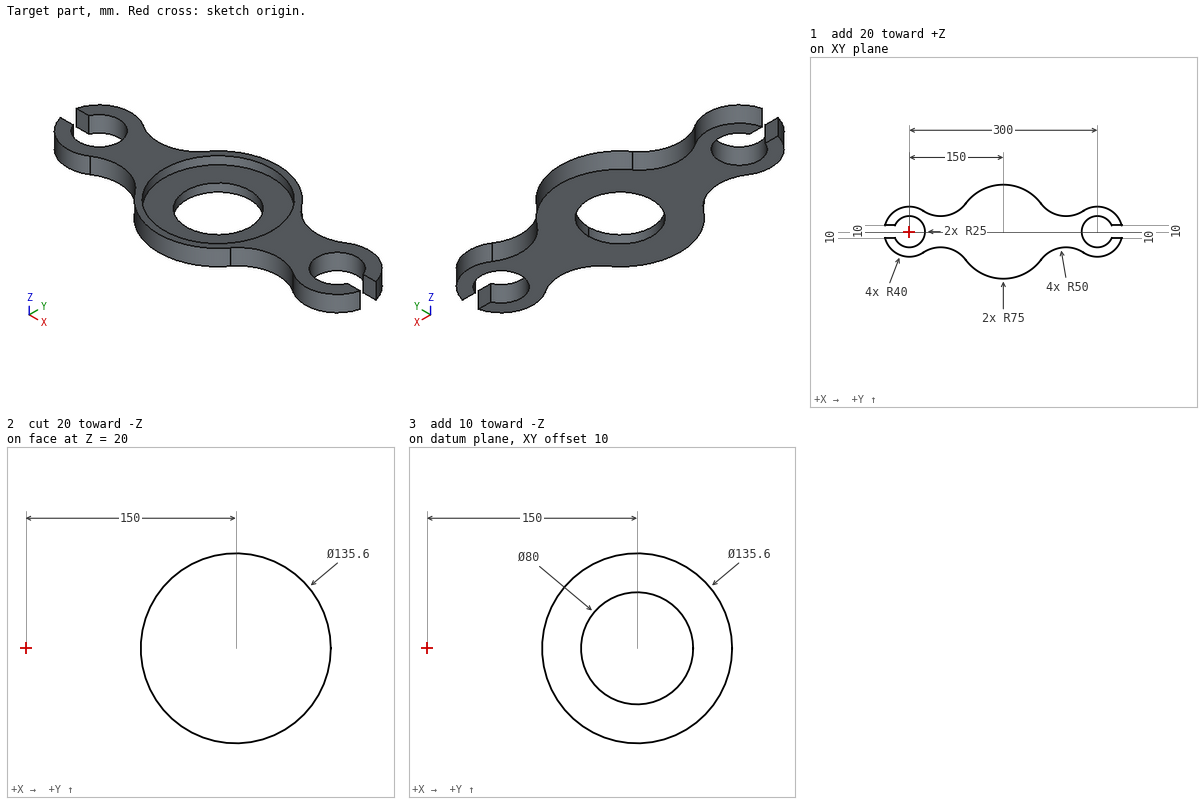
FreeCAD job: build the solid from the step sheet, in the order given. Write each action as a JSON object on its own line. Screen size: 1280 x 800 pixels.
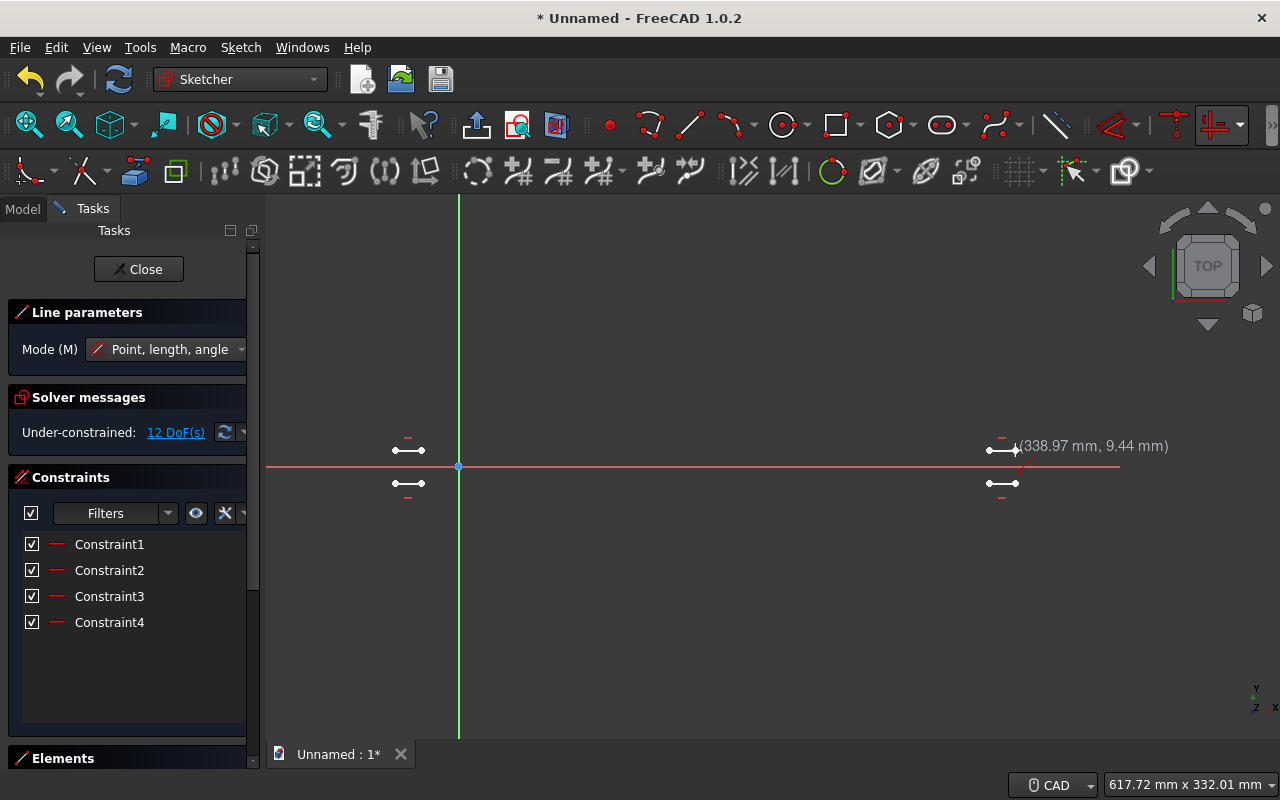
{"action": "left_click", "coordinate": [730, 126]}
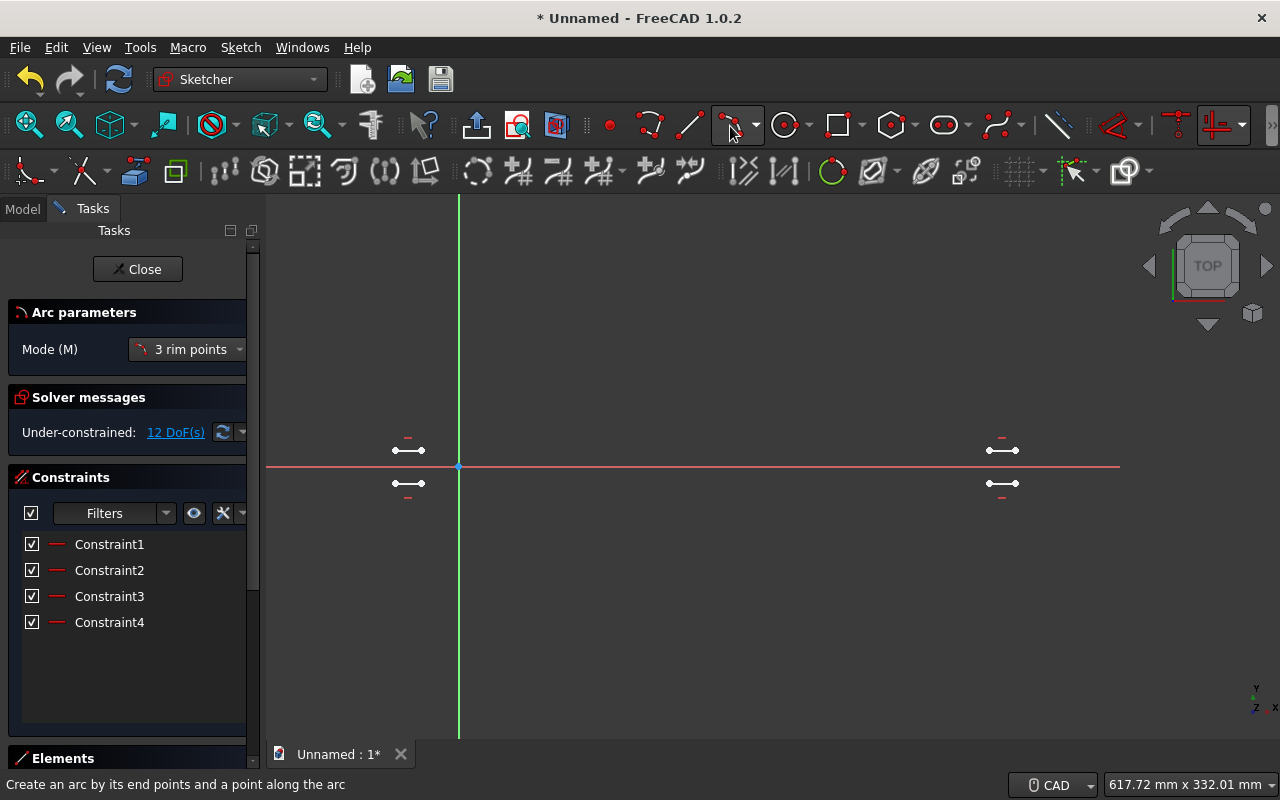
{"action": "scroll", "coordinate": [421, 450], "scroll_direction": "up", "scroll_amount": 2}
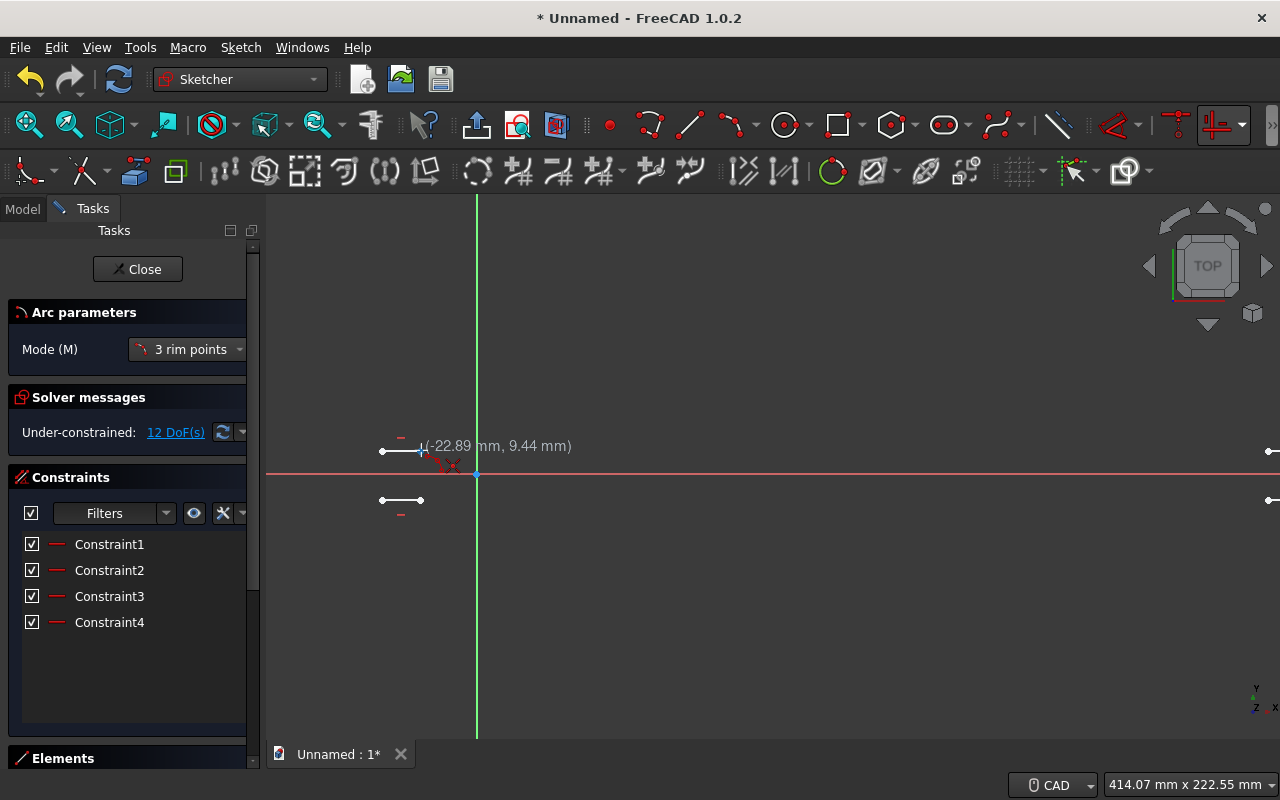
{"action": "left_click", "coordinate": [421, 451]}
{"action": "left_click", "coordinate": [421, 500]}
{"action": "left_click", "coordinate": [529, 506]}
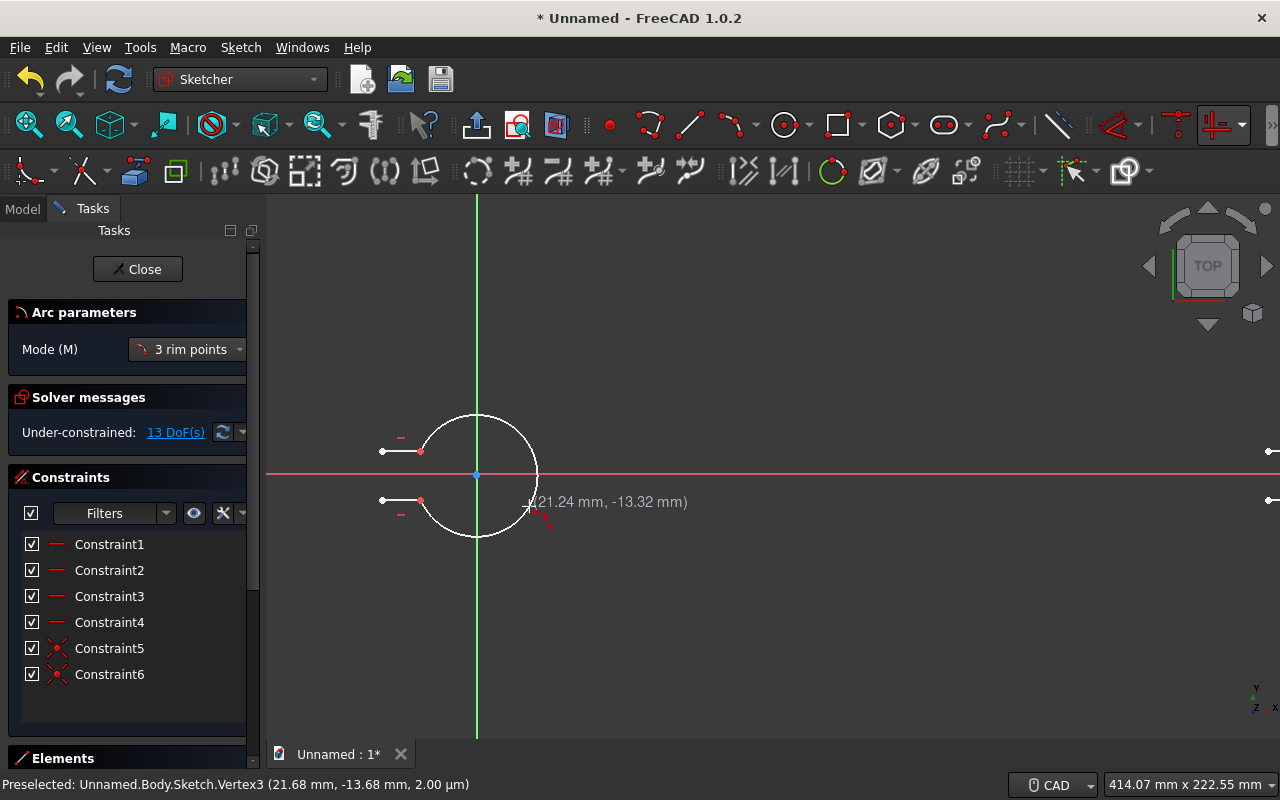
{"action": "left_click", "coordinate": [382, 500]}
{"action": "left_click", "coordinate": [531, 556]}
{"action": "left_click", "coordinate": [442, 566]}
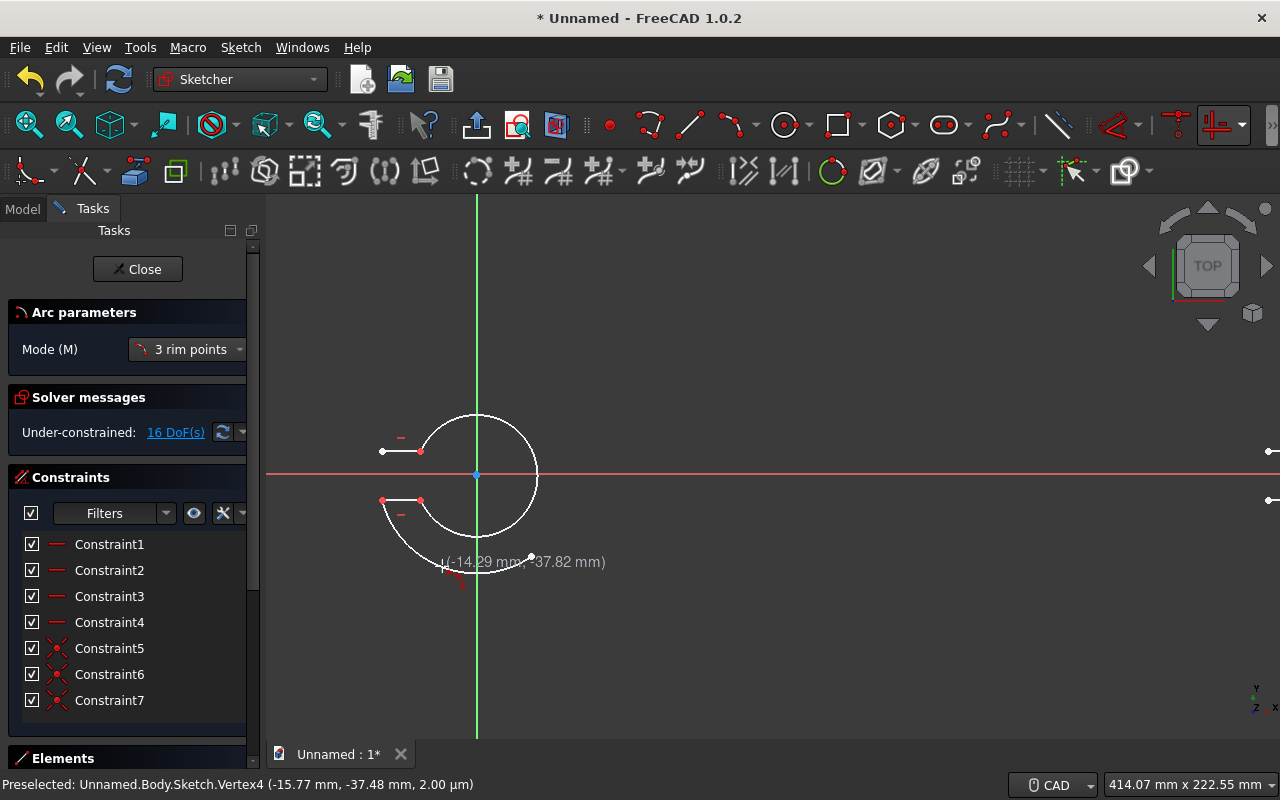
{"action": "left_click", "coordinate": [531, 557]}
{"action": "left_click", "coordinate": [697, 584]}
{"action": "left_click", "coordinate": [620, 537]}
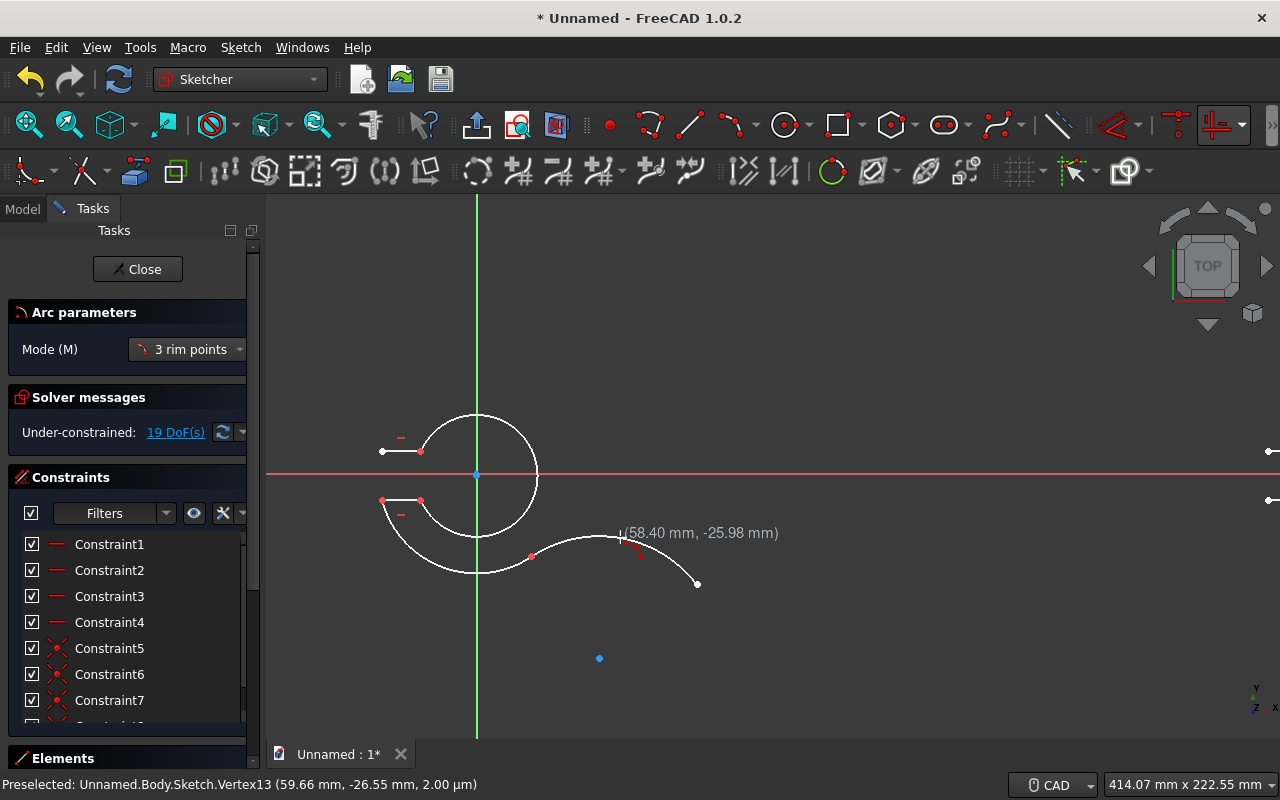
{"action": "left_click", "coordinate": [697, 585]}
{"action": "left_click", "coordinate": [991, 584]}
{"action": "left_click", "coordinate": [844, 658]}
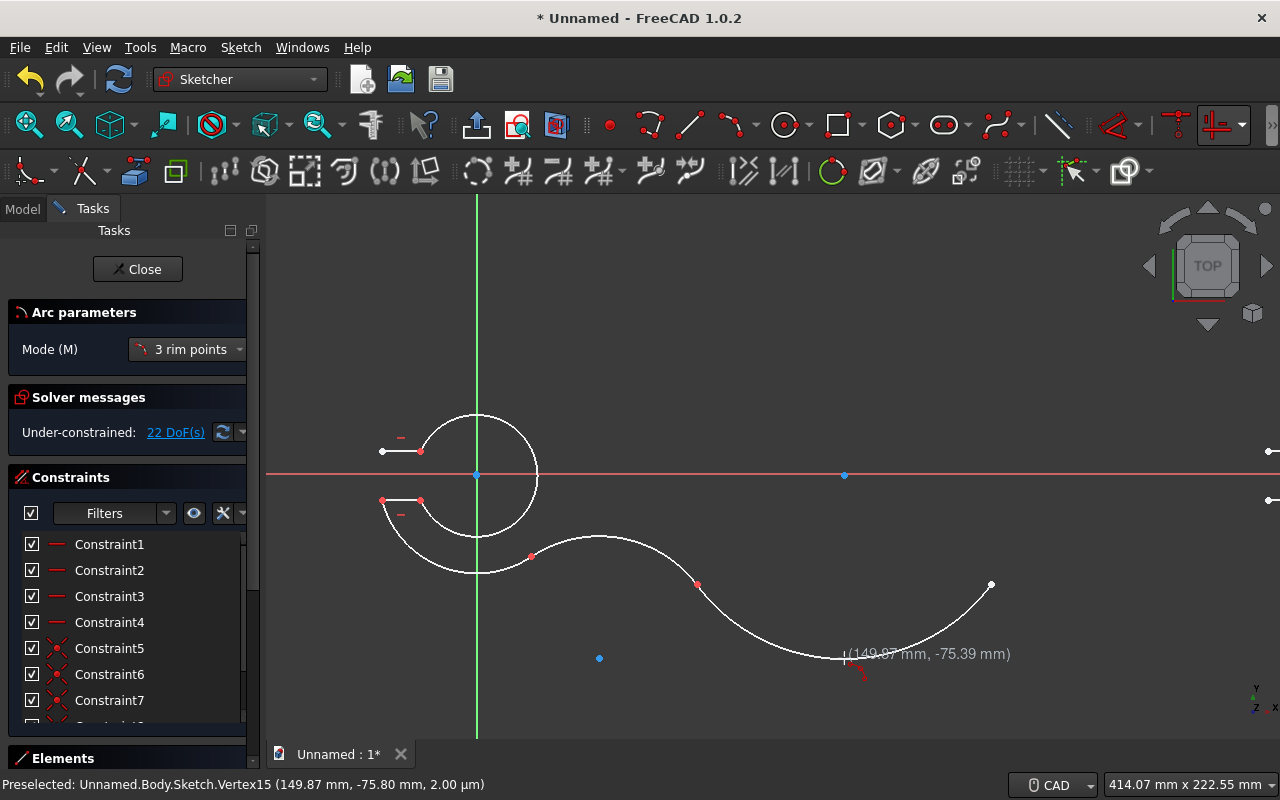
{"action": "left_click", "coordinate": [991, 585]}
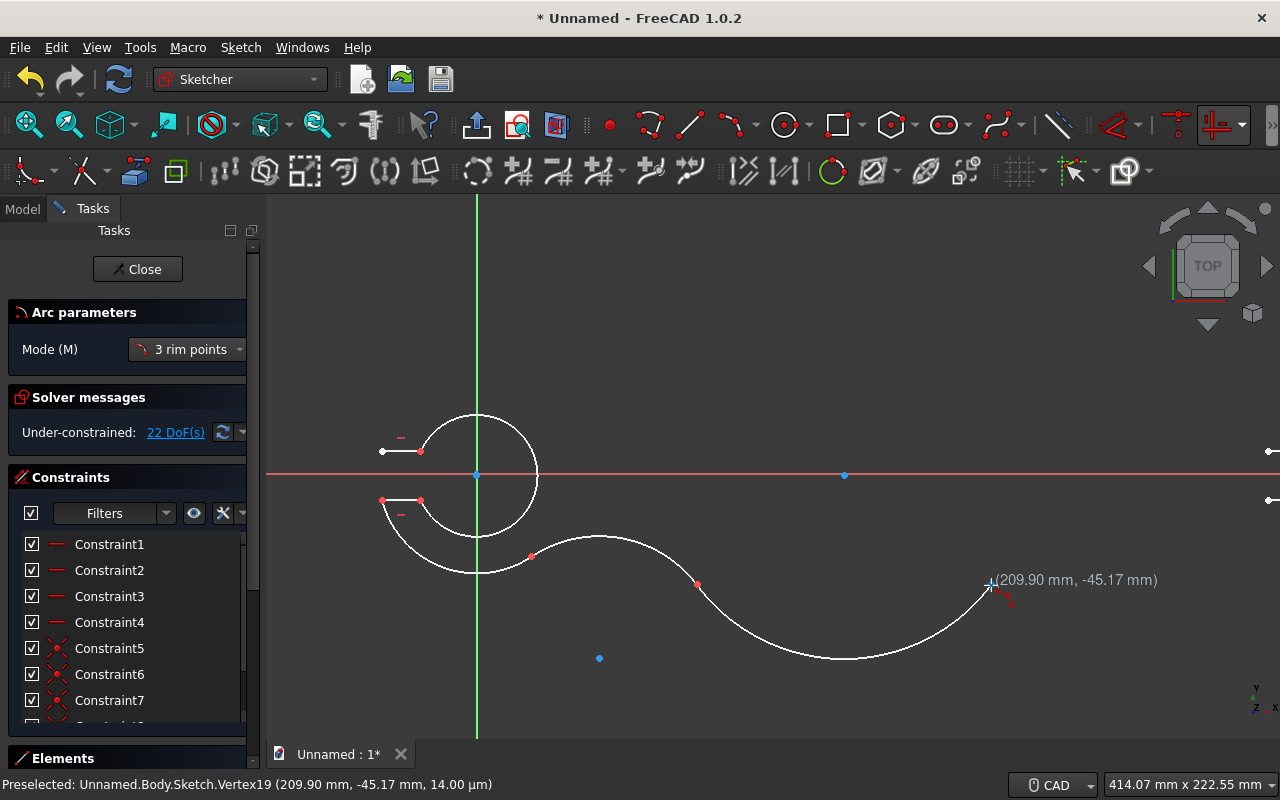
{"action": "scroll", "coordinate": [420, 450], "scroll_direction": "down", "scroll_amount": 2}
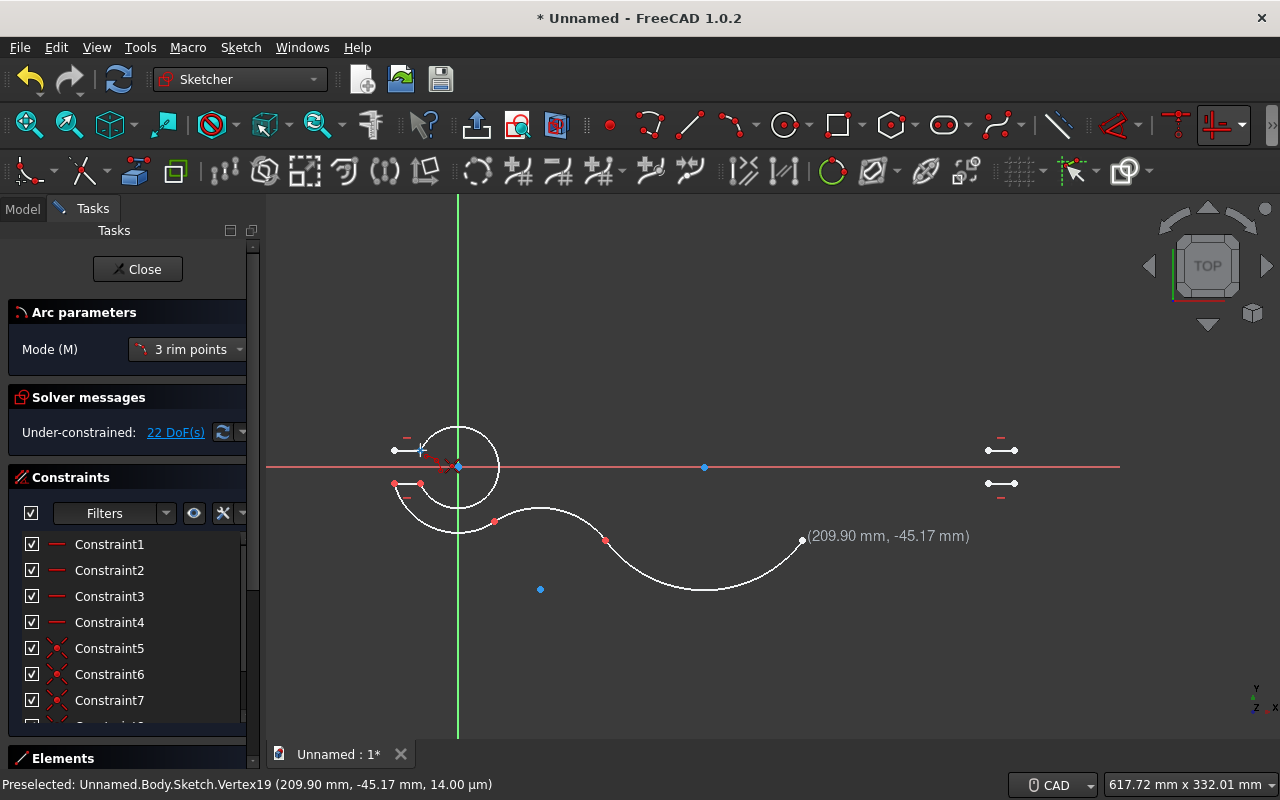
{"action": "left_click", "coordinate": [914, 521]}
{"action": "left_click", "coordinate": [855, 509]}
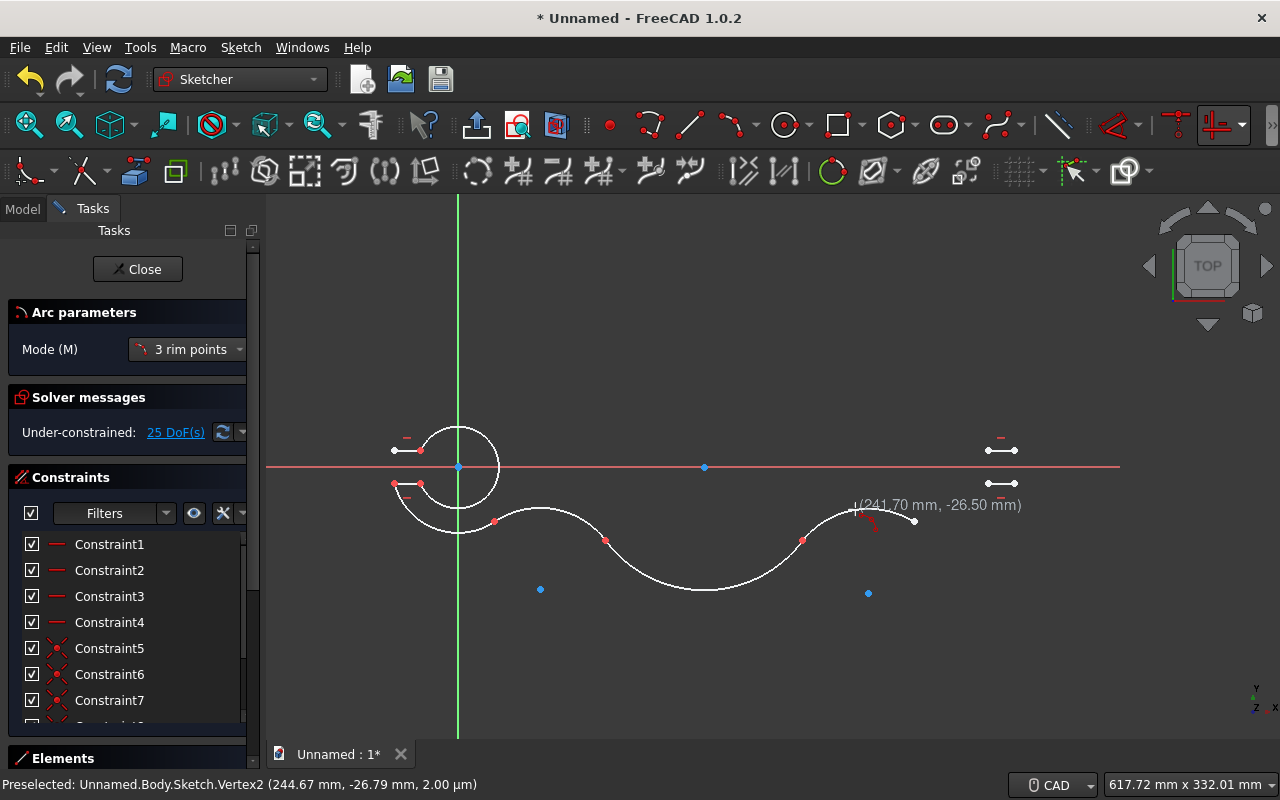
{"action": "left_click", "coordinate": [914, 522]}